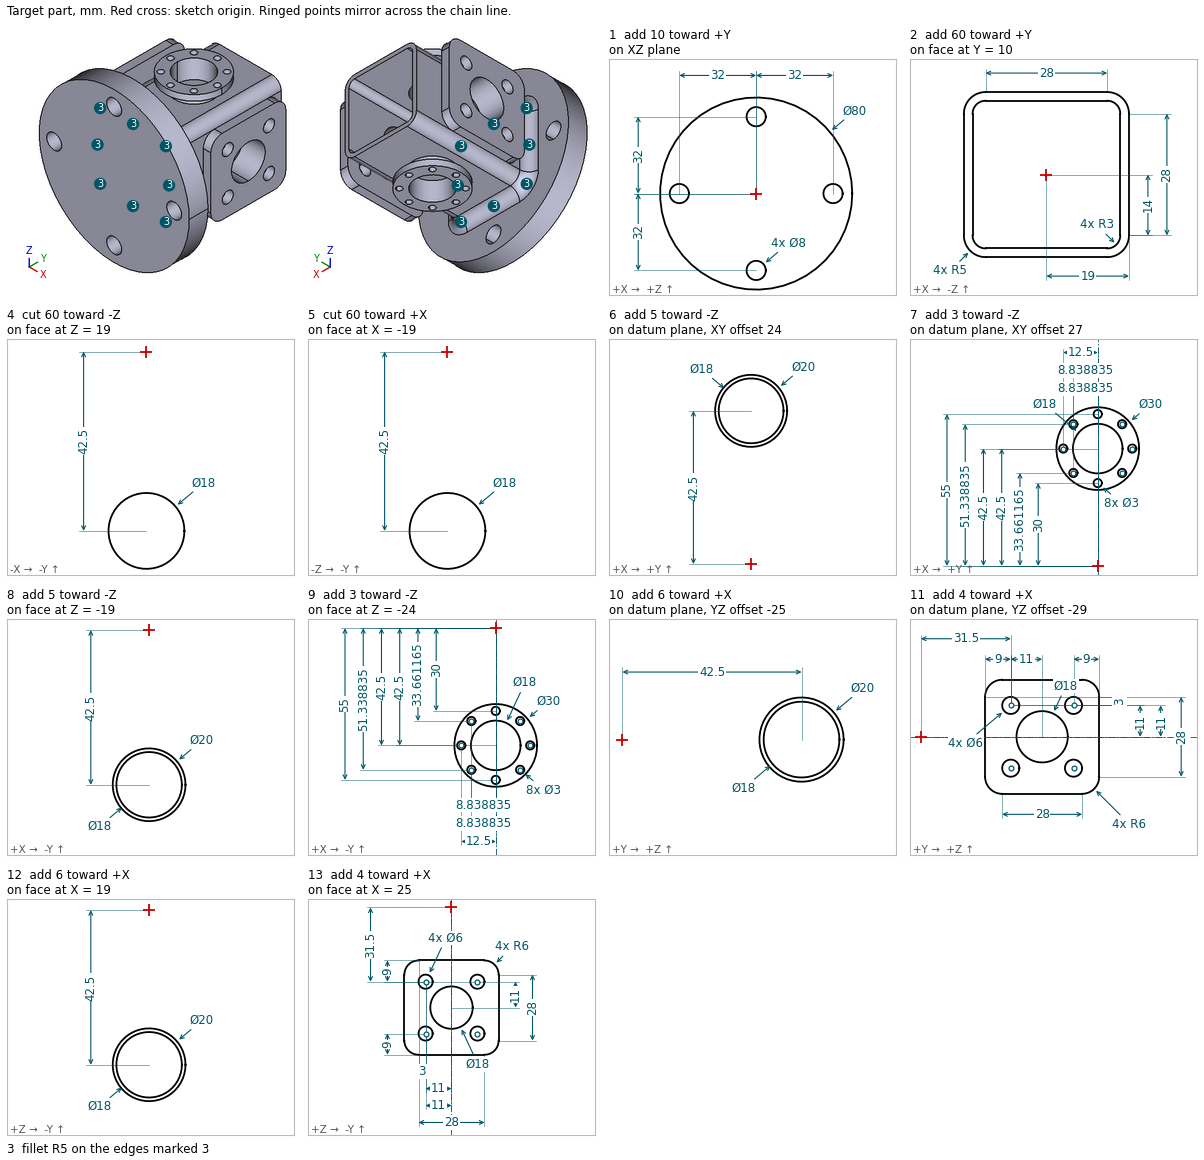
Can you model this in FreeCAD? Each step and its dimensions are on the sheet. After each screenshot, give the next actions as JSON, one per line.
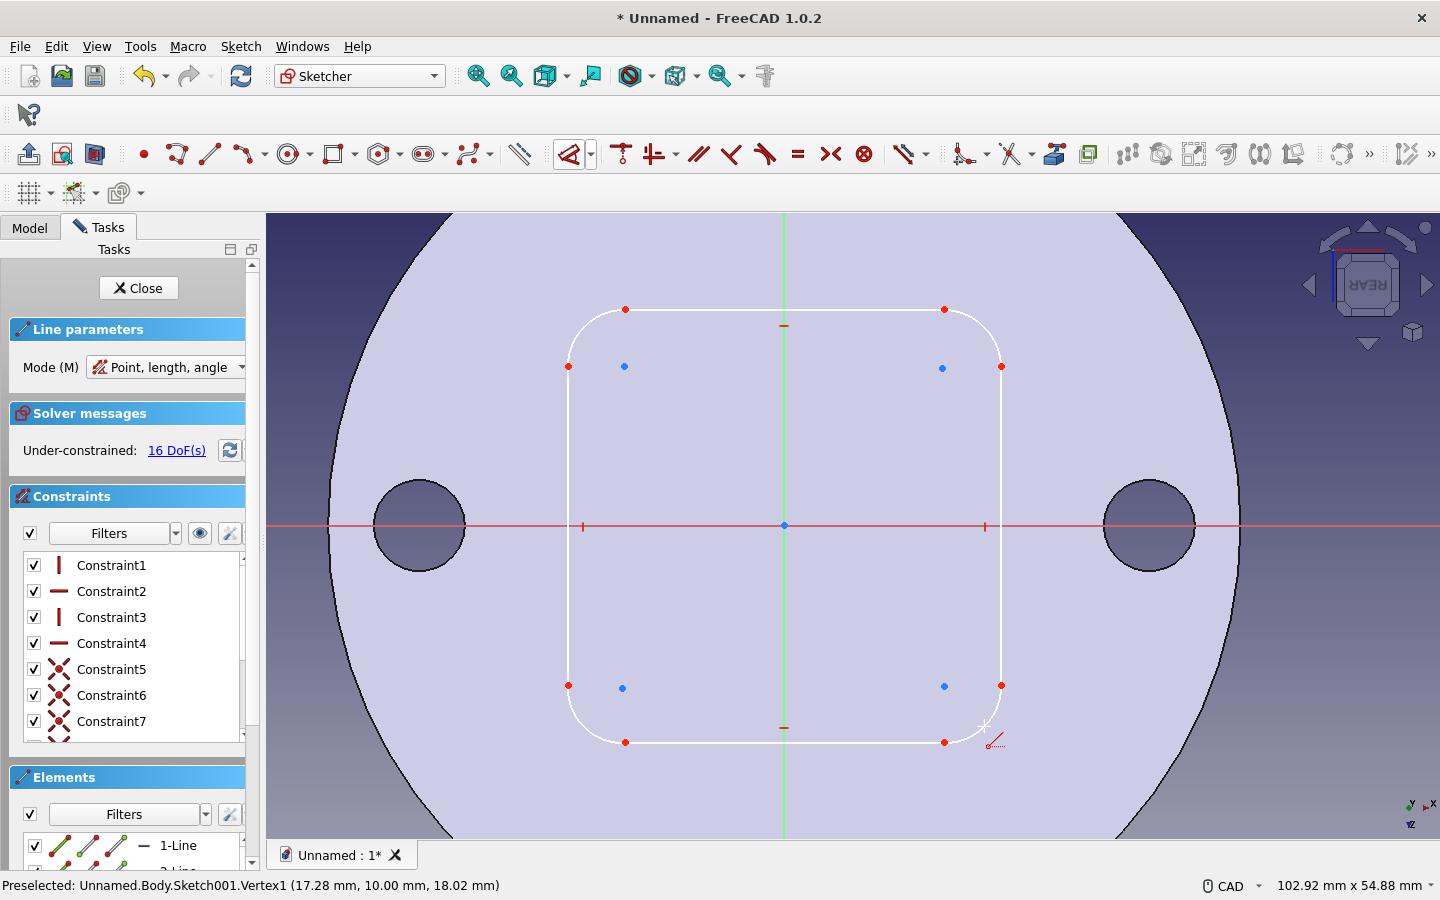
{"action": "left_click", "coordinate": [978, 366]}
{"action": "left_click", "coordinate": [978, 685]}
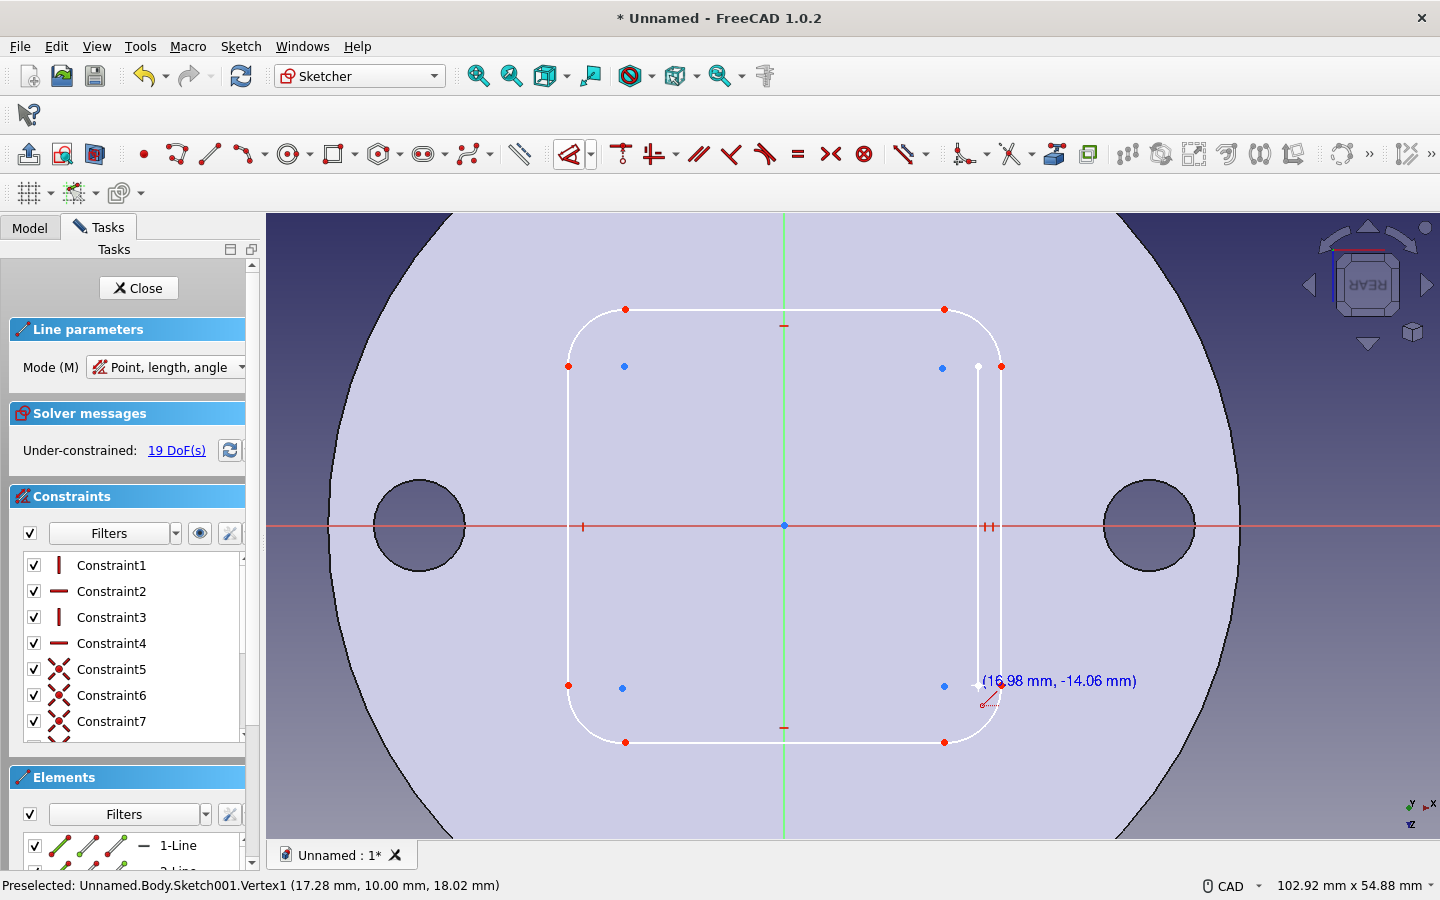
{"action": "left_click", "coordinate": [944, 719]}
{"action": "left_click", "coordinate": [625, 719]}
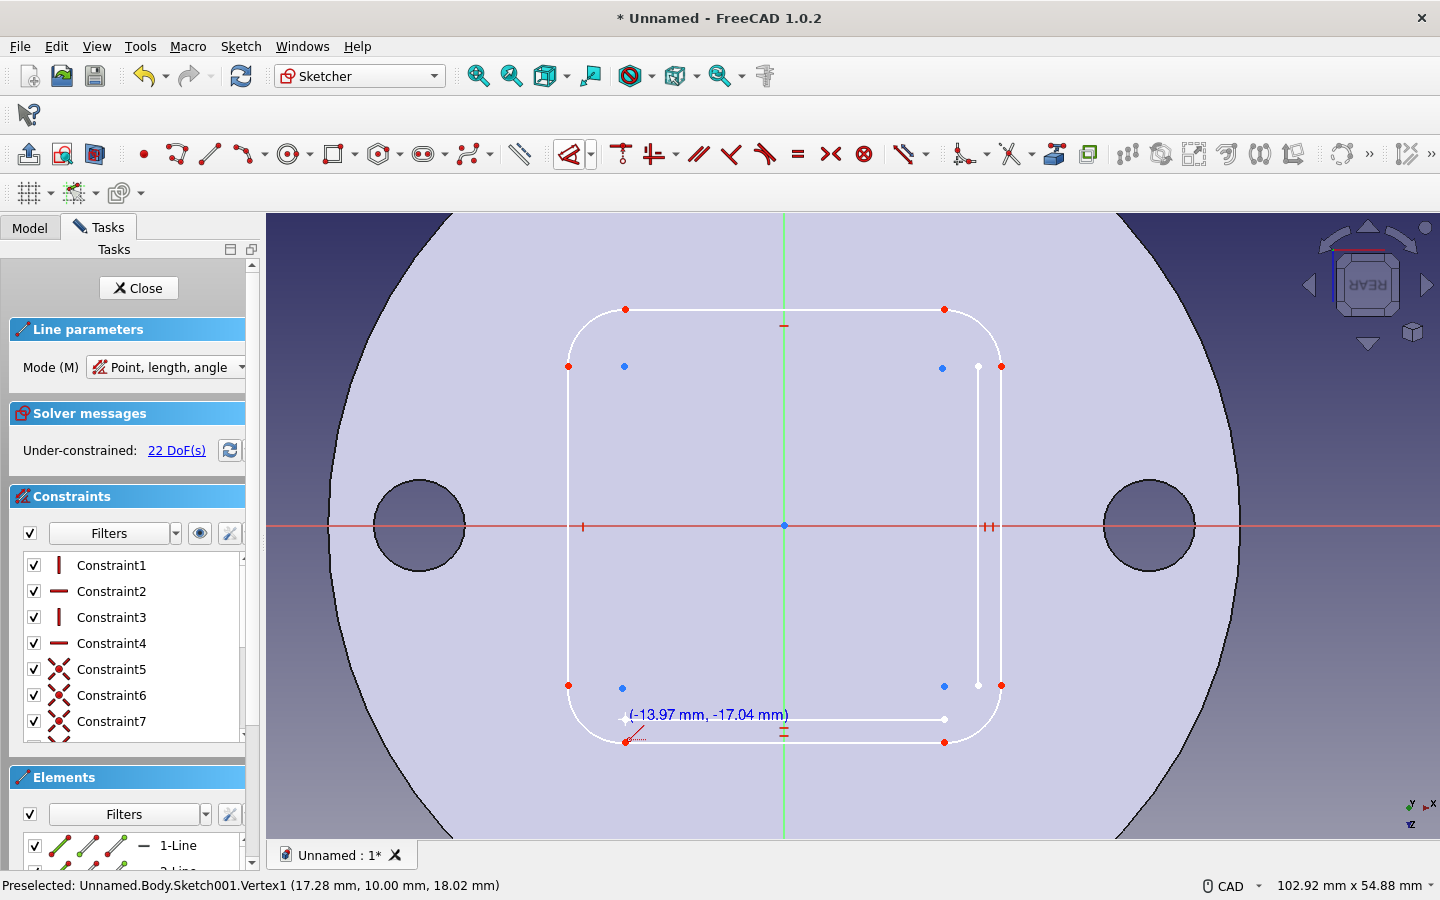
{"action": "left_click", "coordinate": [590, 685]}
{"action": "left_click", "coordinate": [590, 366]}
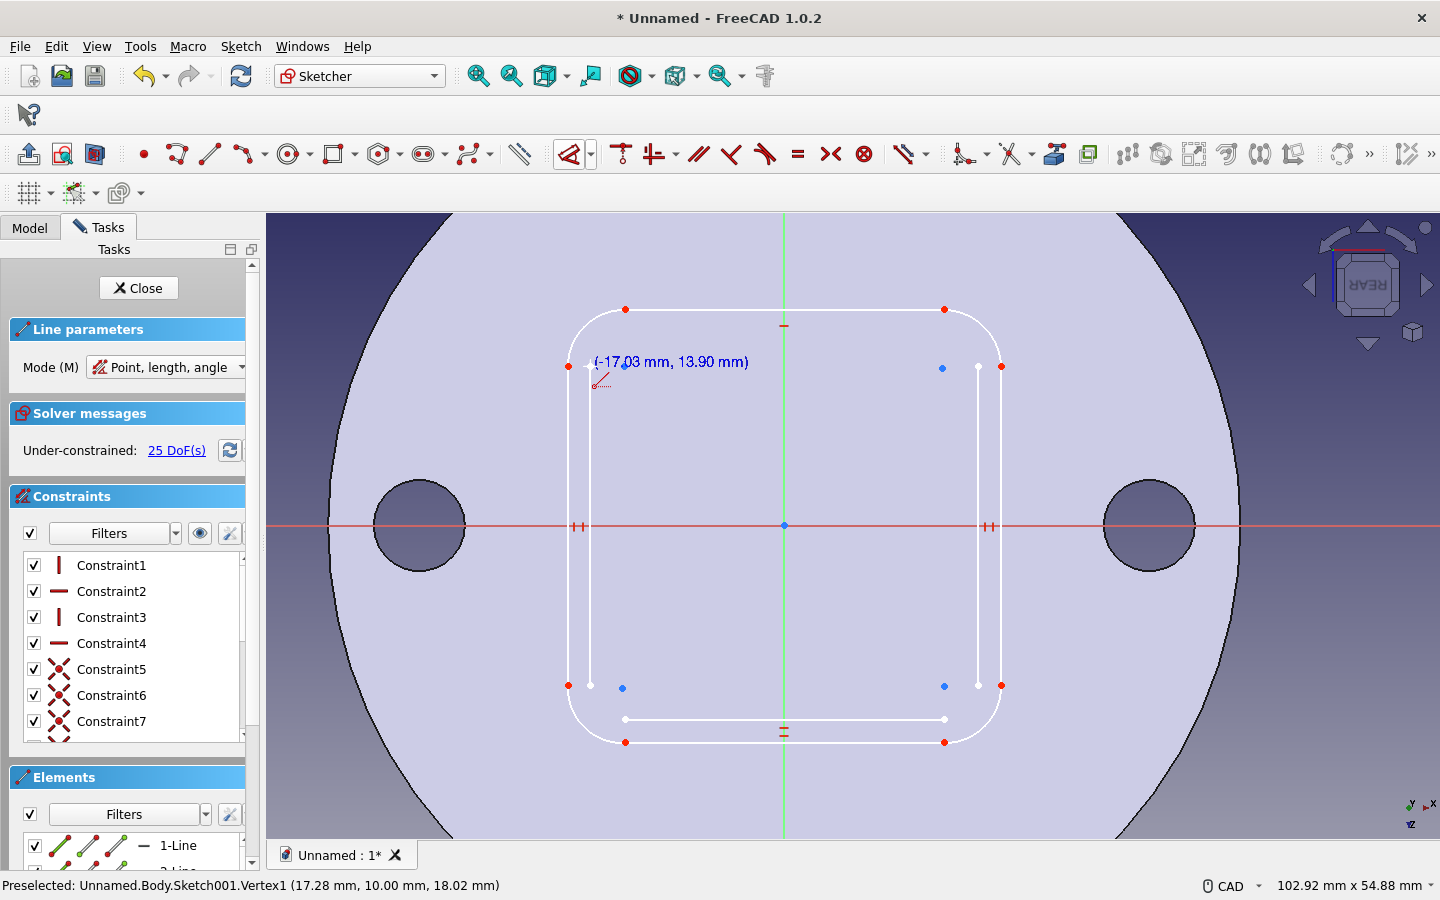
{"action": "left_click", "coordinate": [625, 332]}
{"action": "left_click", "coordinate": [944, 332]}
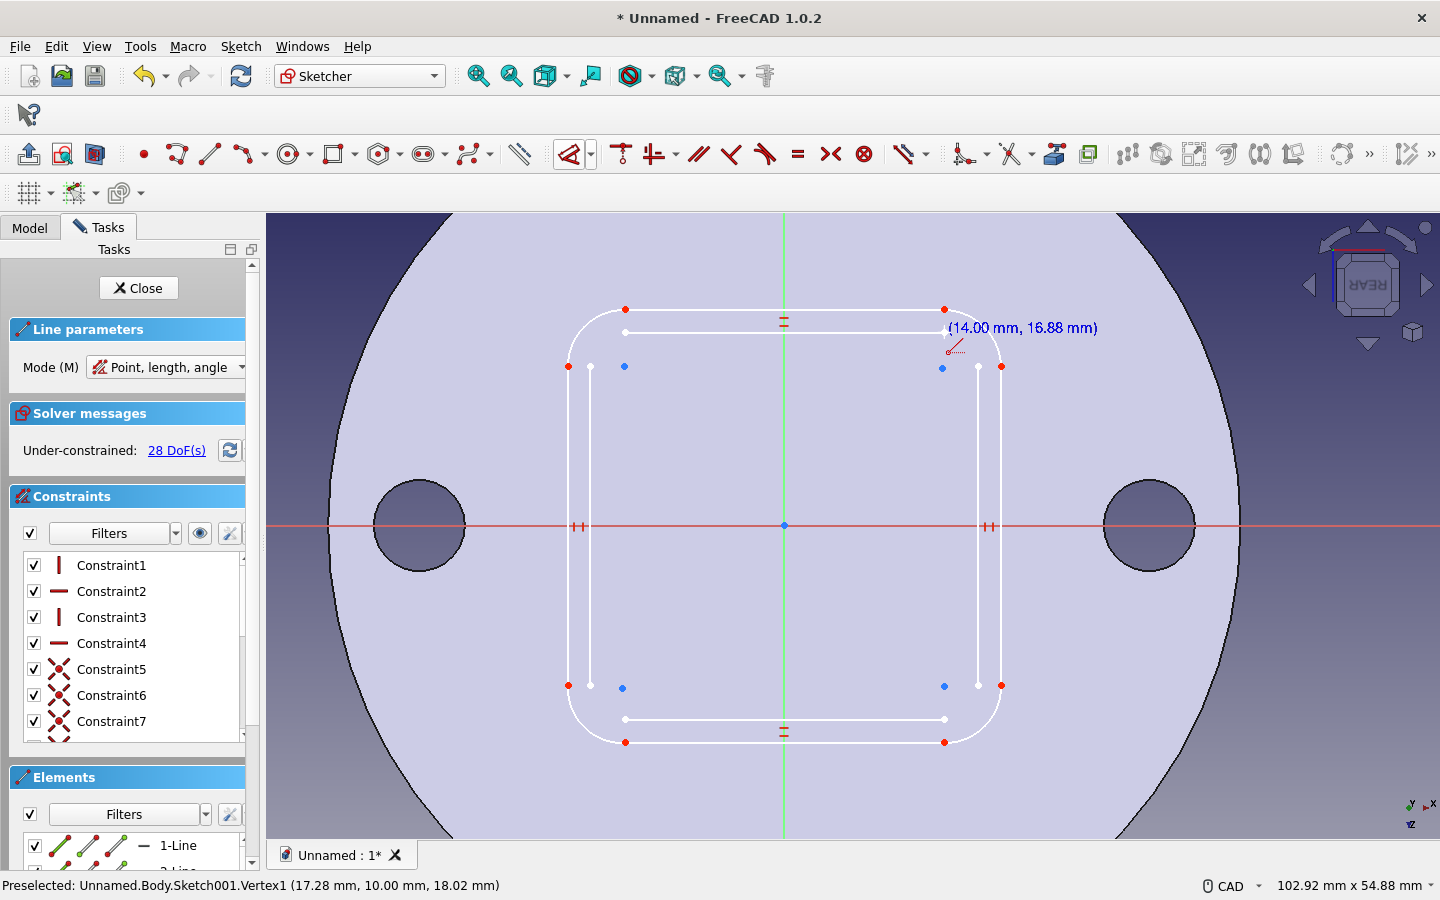
{"action": "key", "text": "g 3 a"}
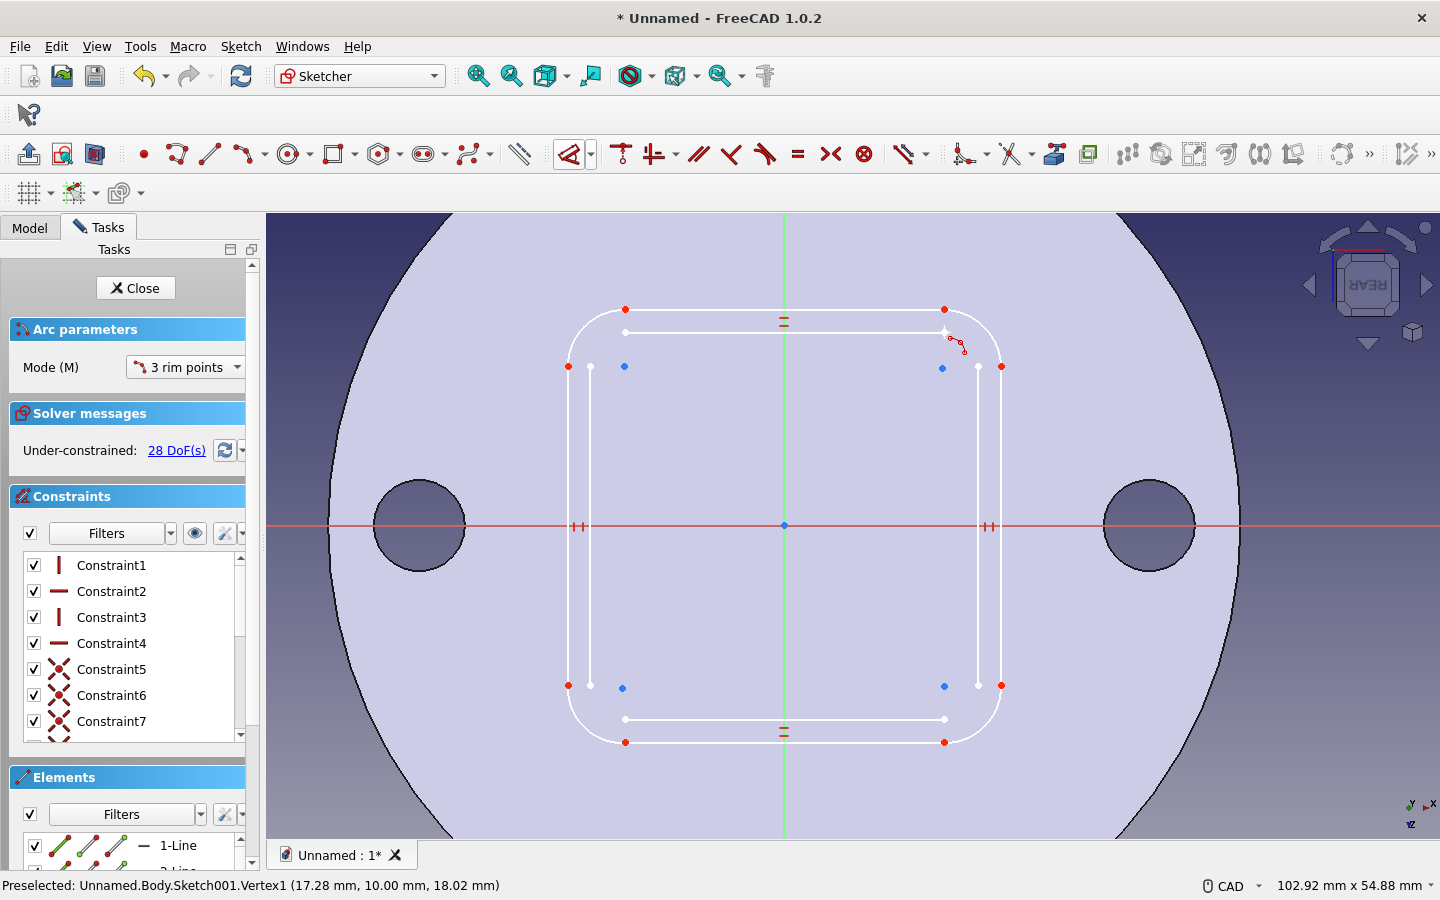
{"action": "left_click", "coordinate": [978, 686]}
{"action": "left_click", "coordinate": [944, 720]}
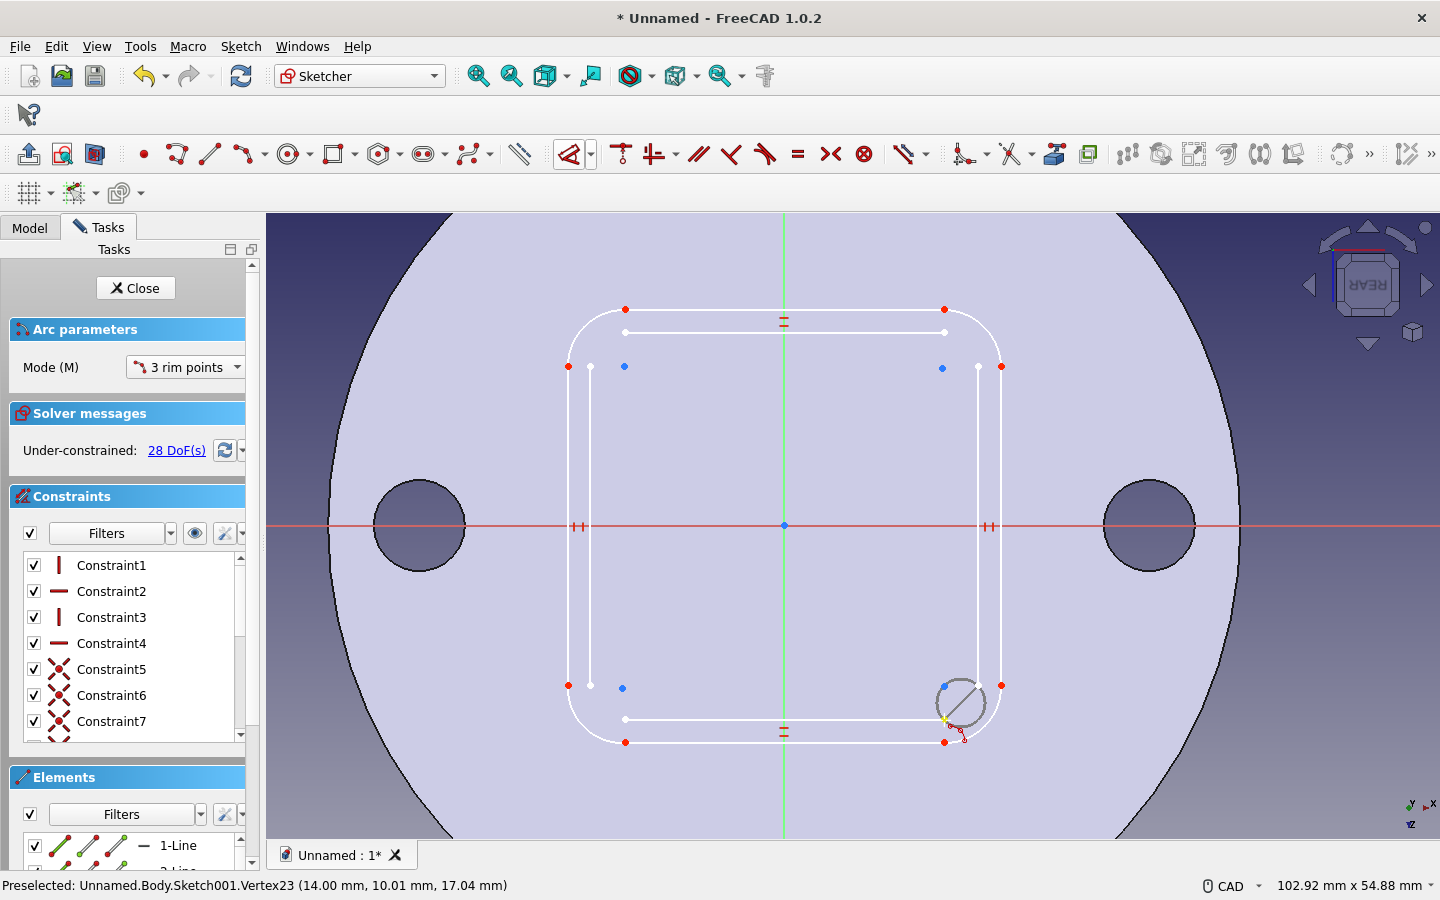
{"action": "scroll", "coordinate": [968, 709], "scroll_direction": "up", "scroll_amount": 3}